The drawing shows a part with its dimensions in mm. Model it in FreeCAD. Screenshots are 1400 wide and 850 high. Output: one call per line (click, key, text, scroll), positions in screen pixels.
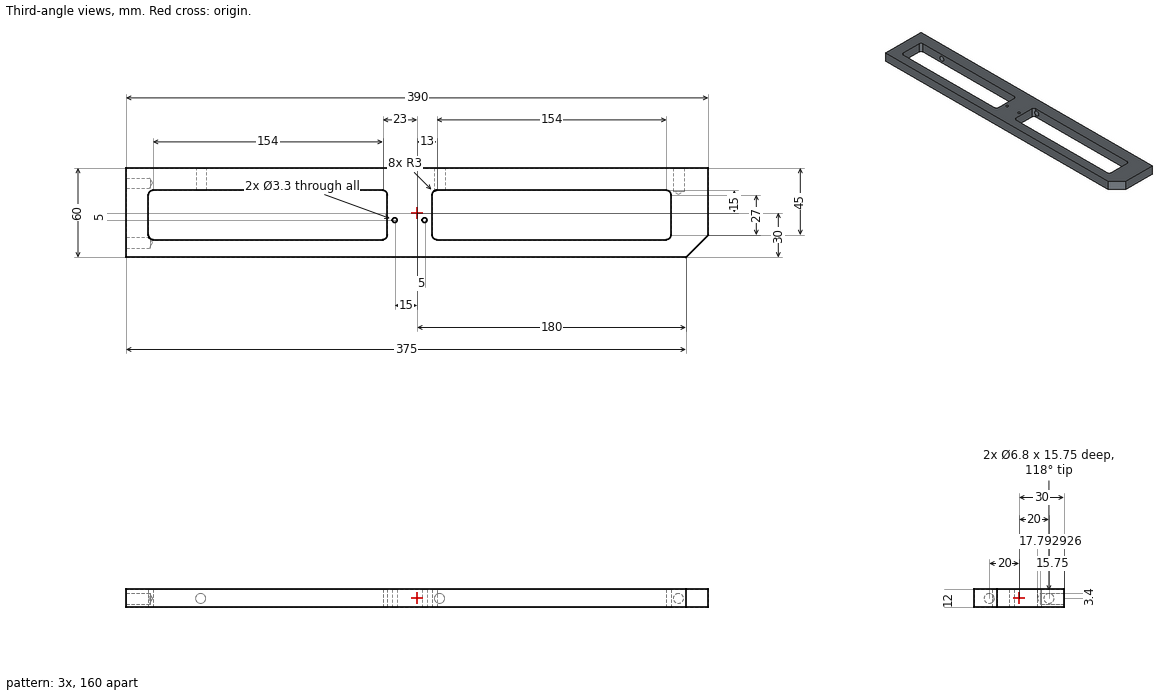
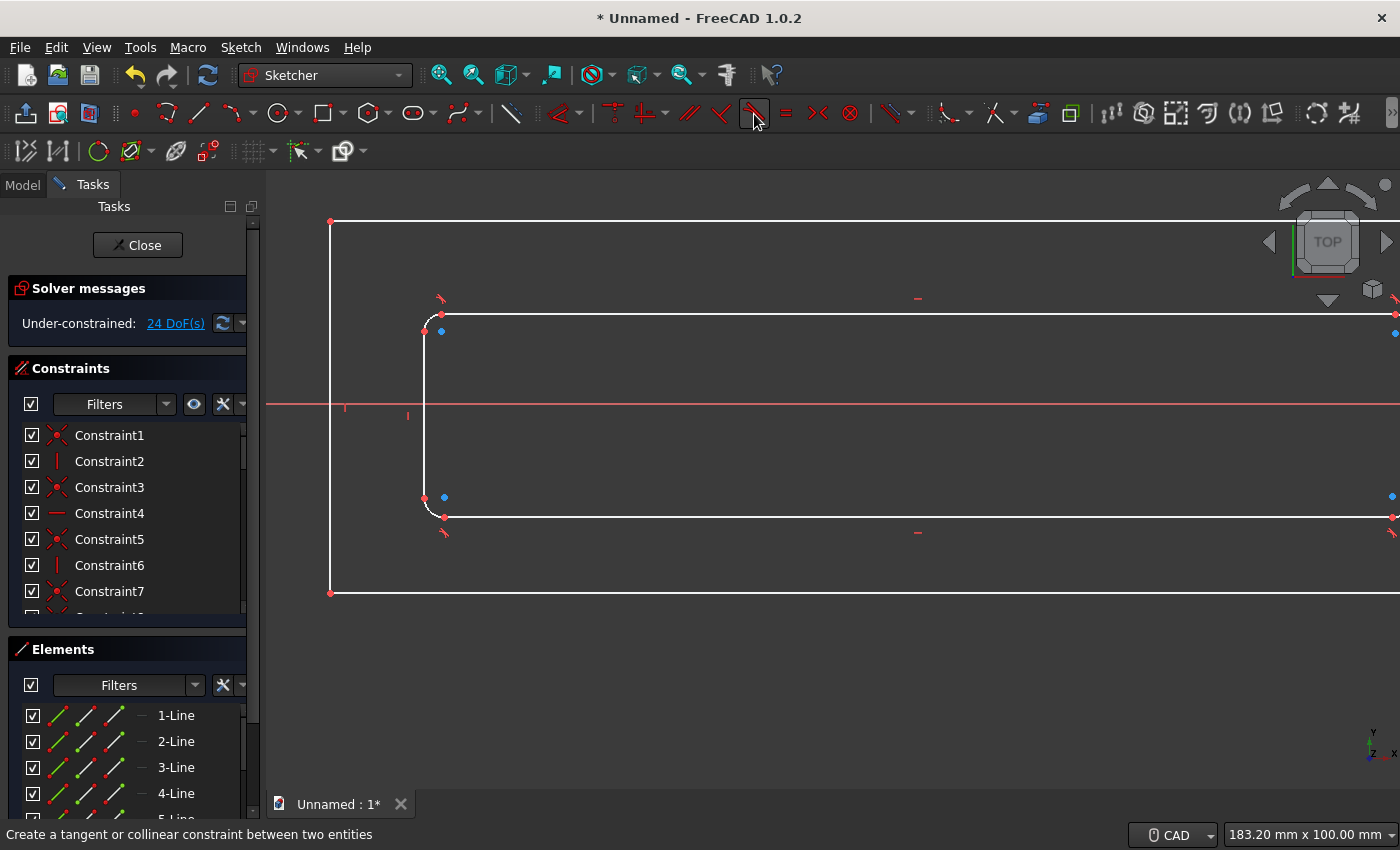
click(424, 449)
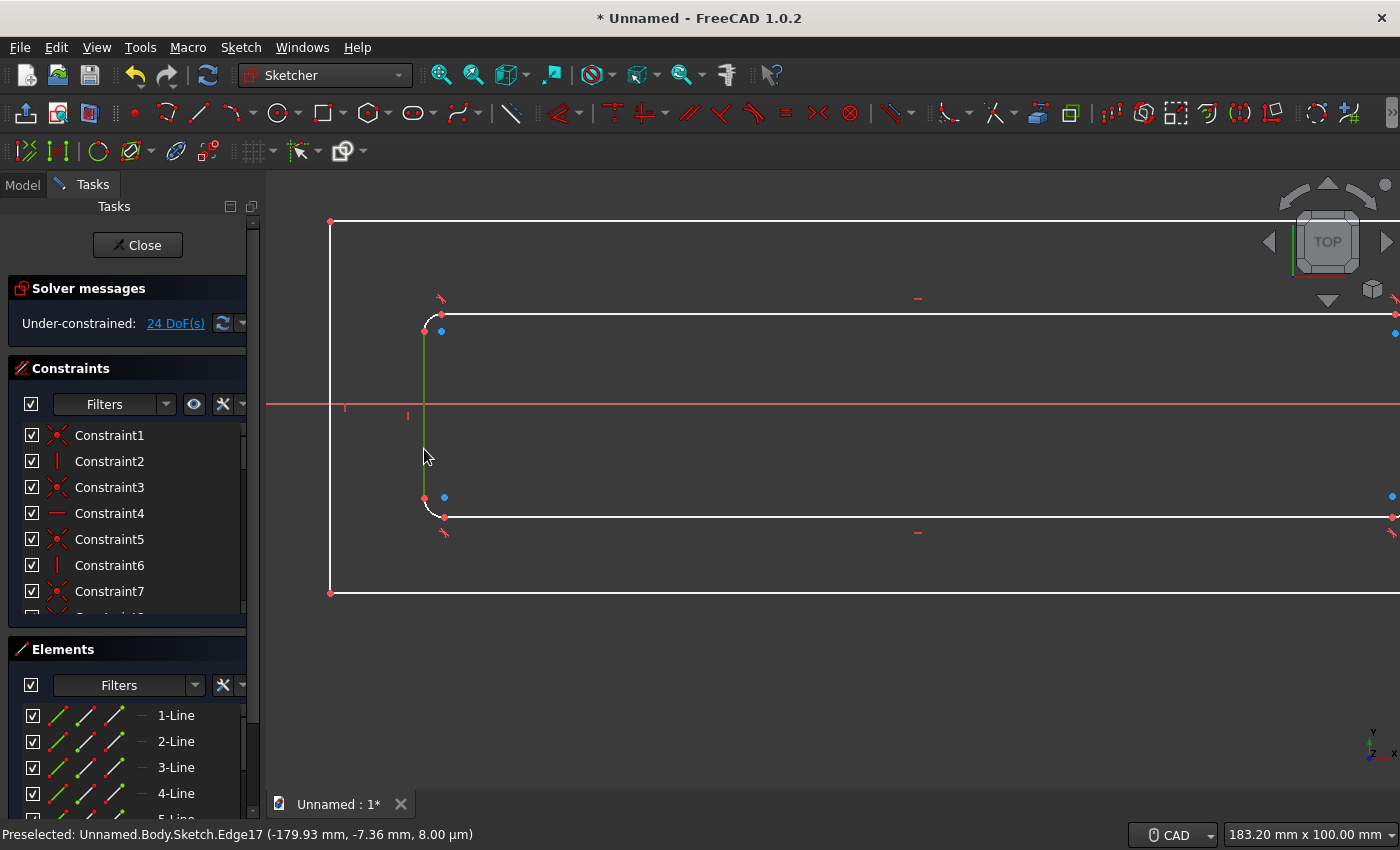
click(431, 512)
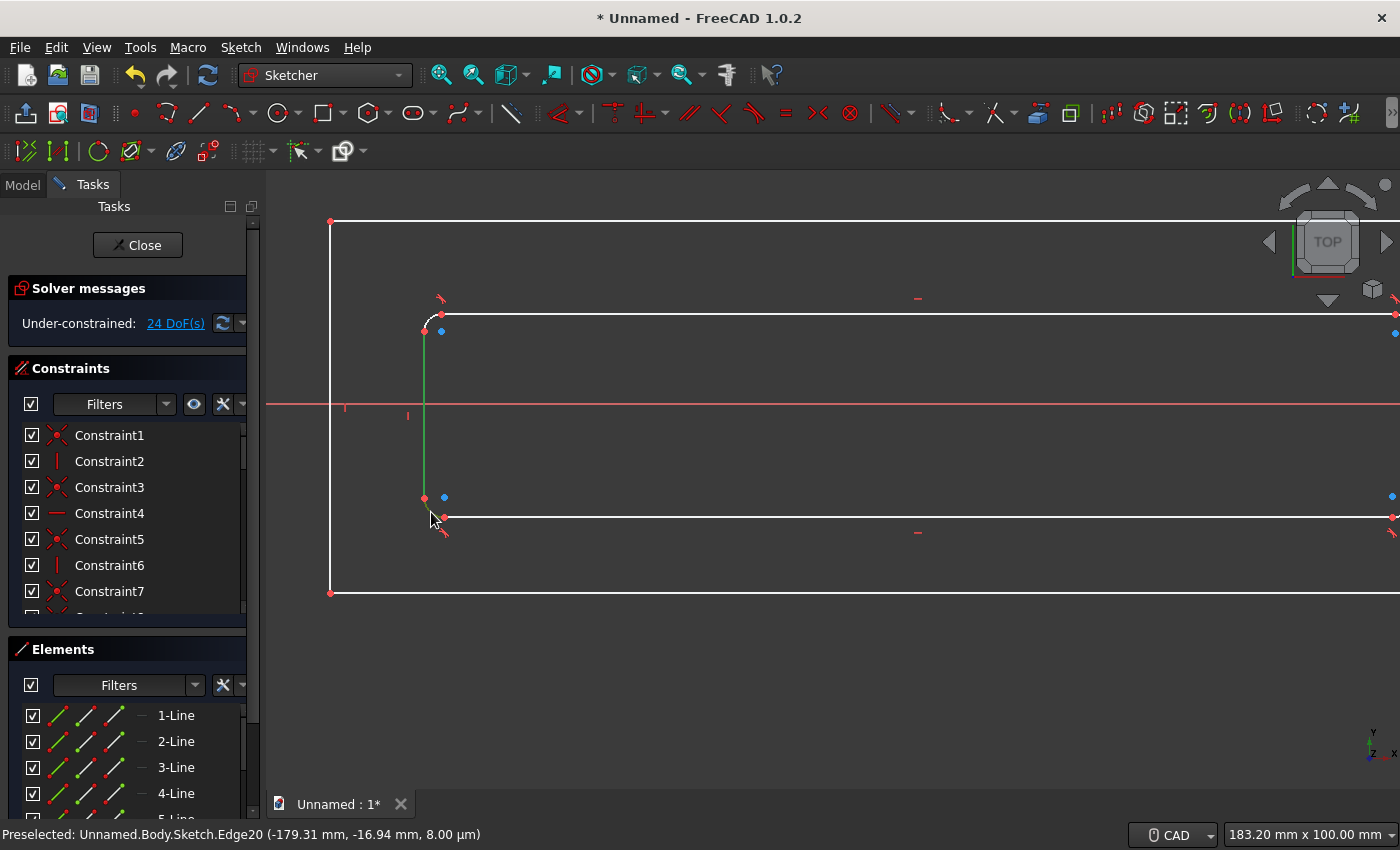
click(754, 114)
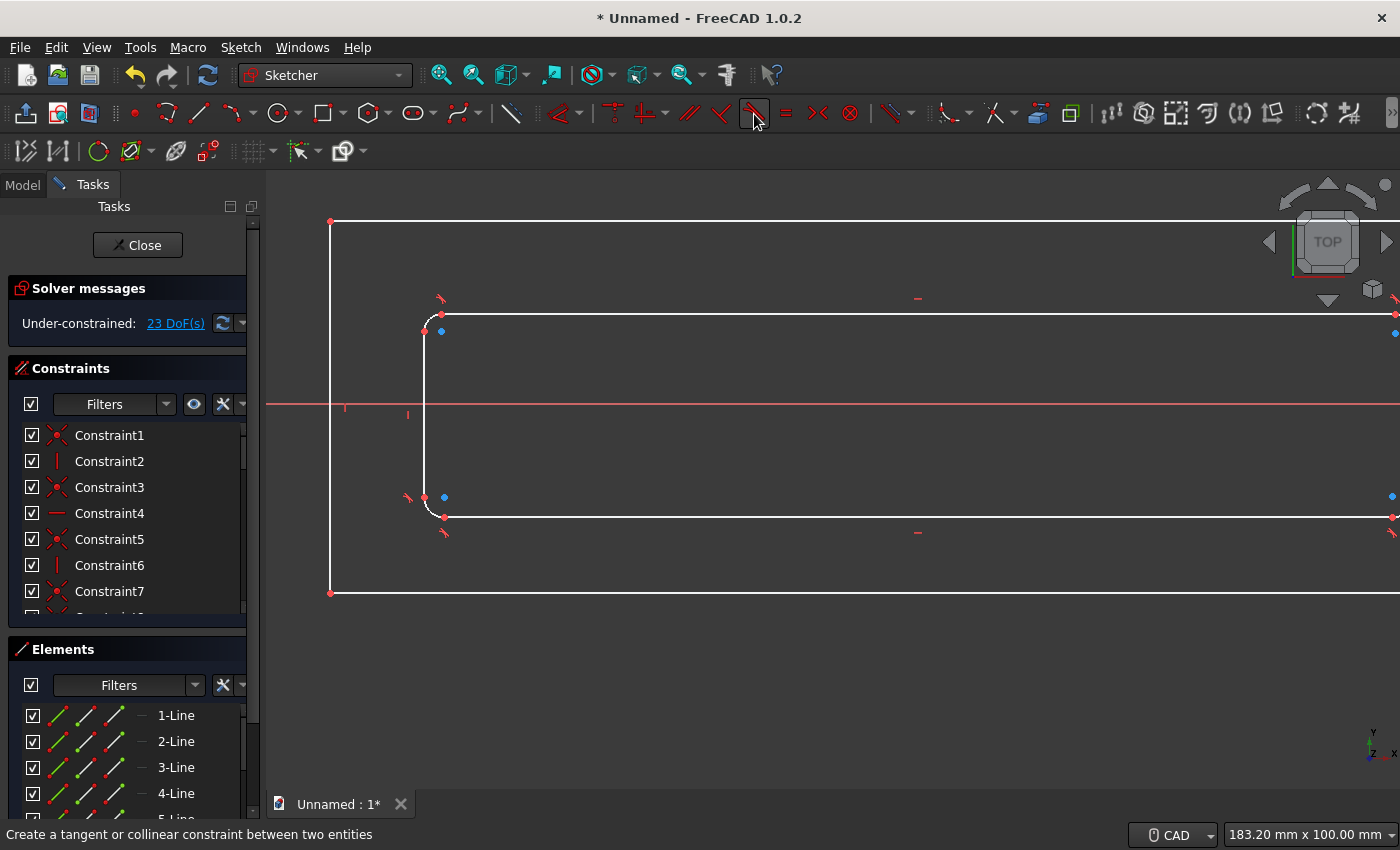
click(424, 448)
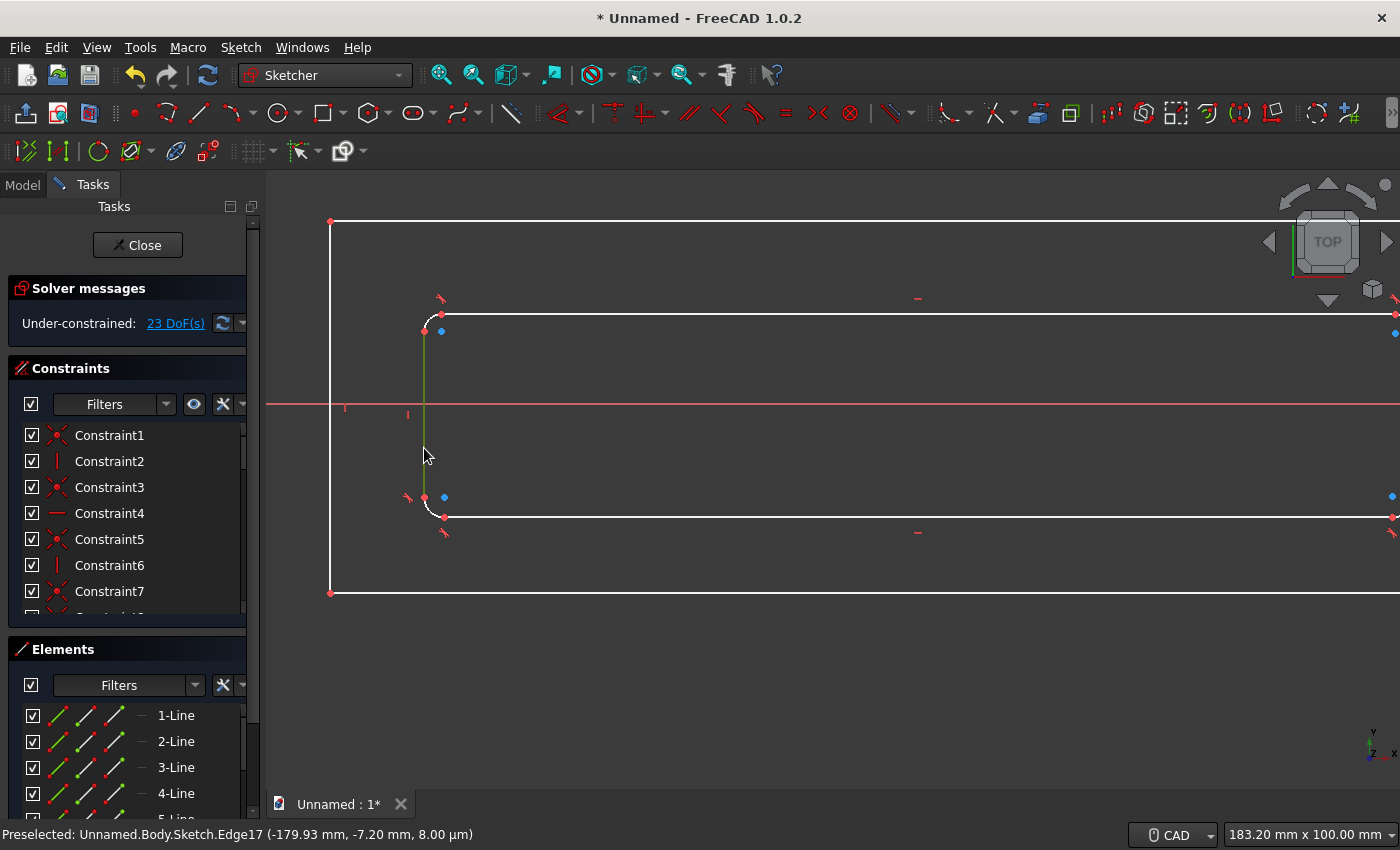
click(429, 319)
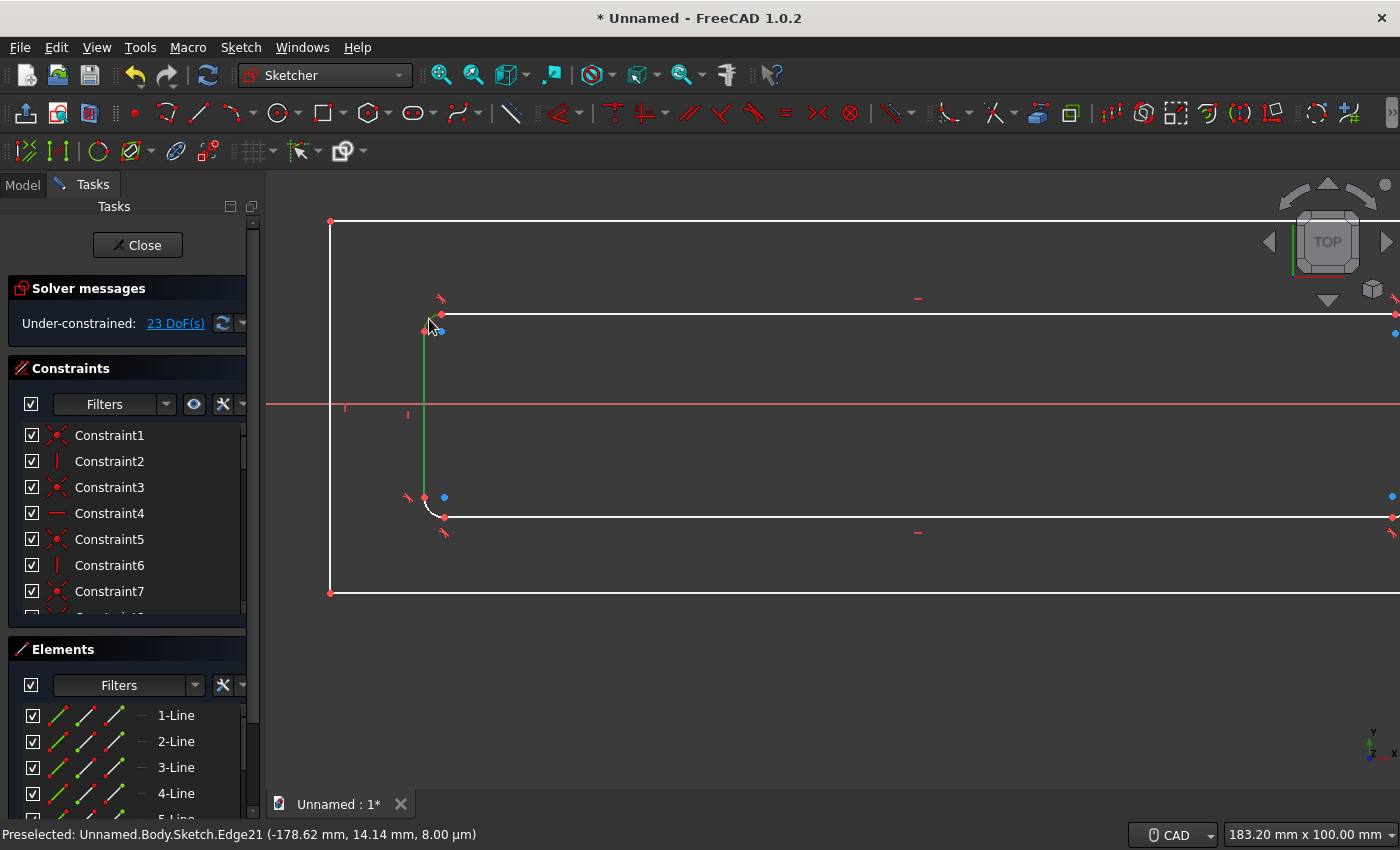
click(754, 114)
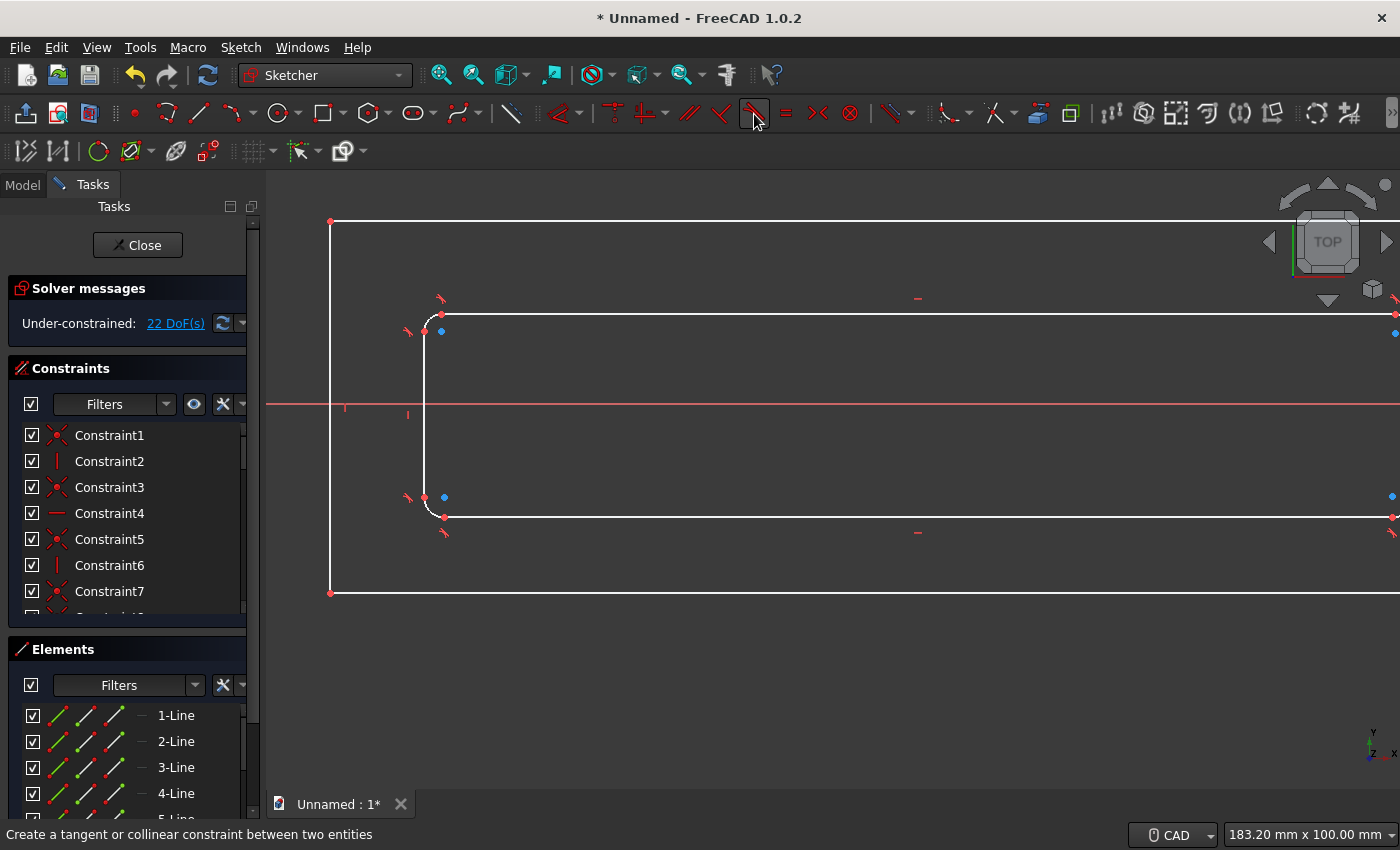
scroll(431, 512, down, 6)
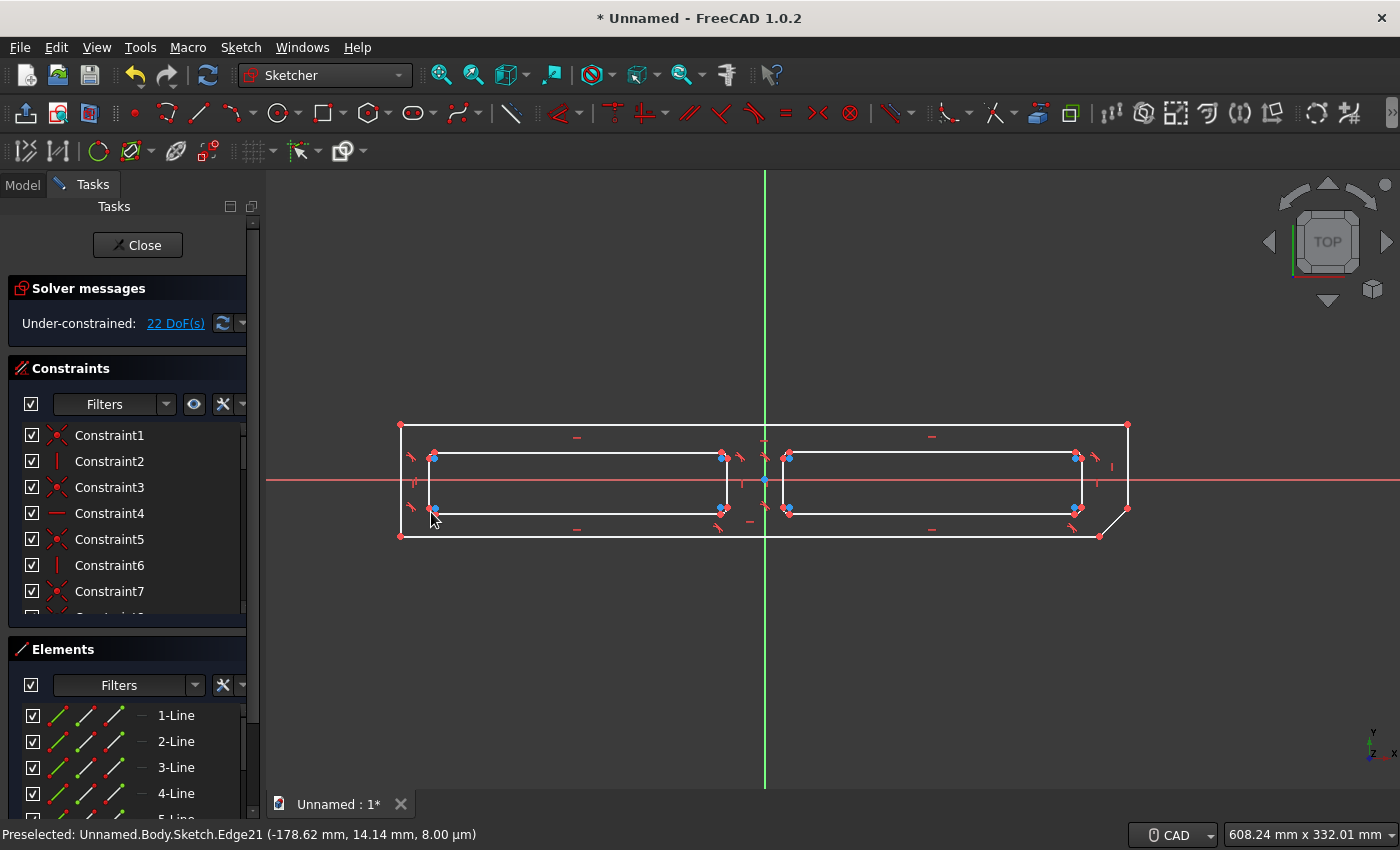
scroll(1081, 455, up, 9)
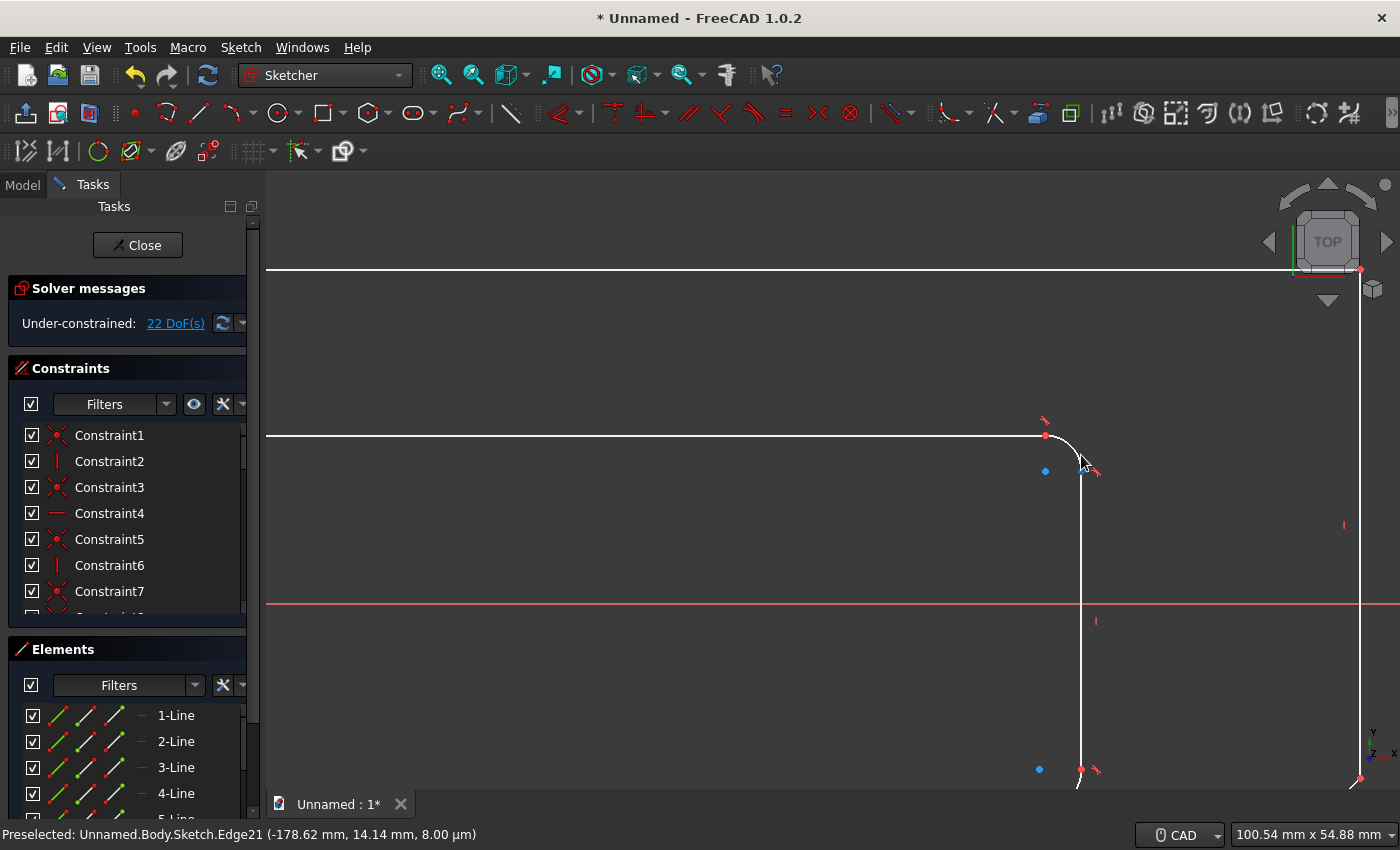
click(1077, 455)